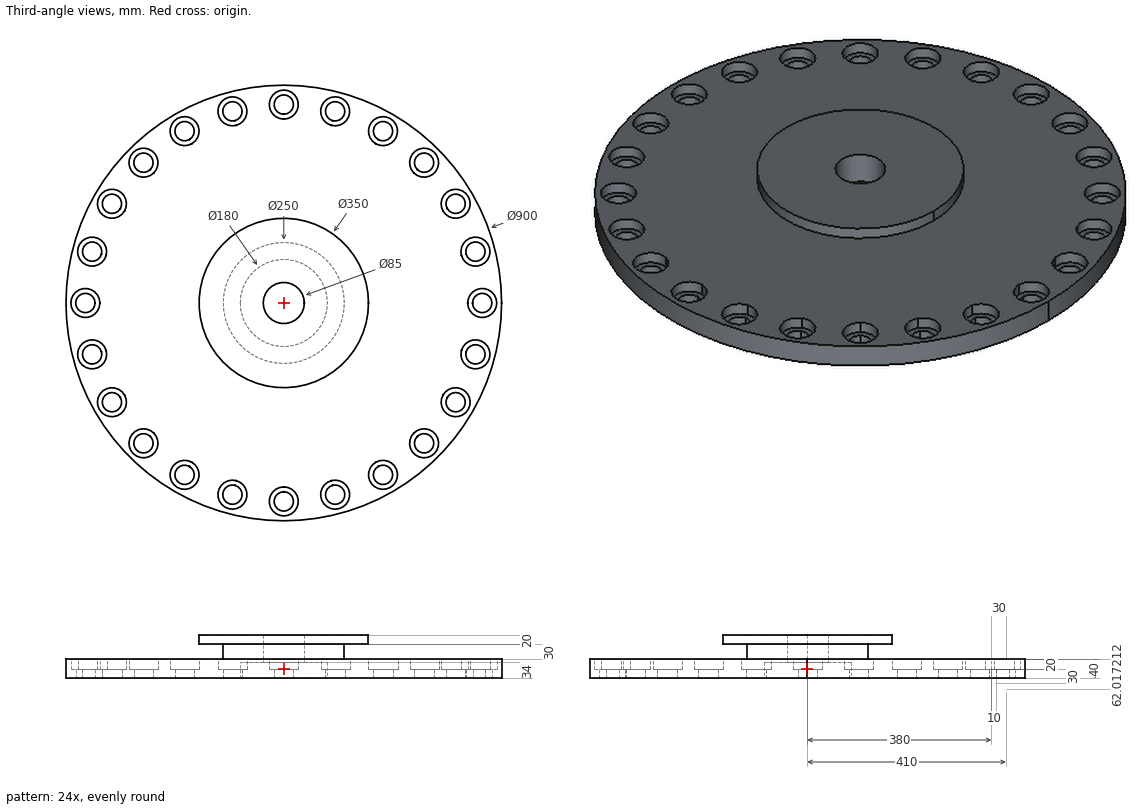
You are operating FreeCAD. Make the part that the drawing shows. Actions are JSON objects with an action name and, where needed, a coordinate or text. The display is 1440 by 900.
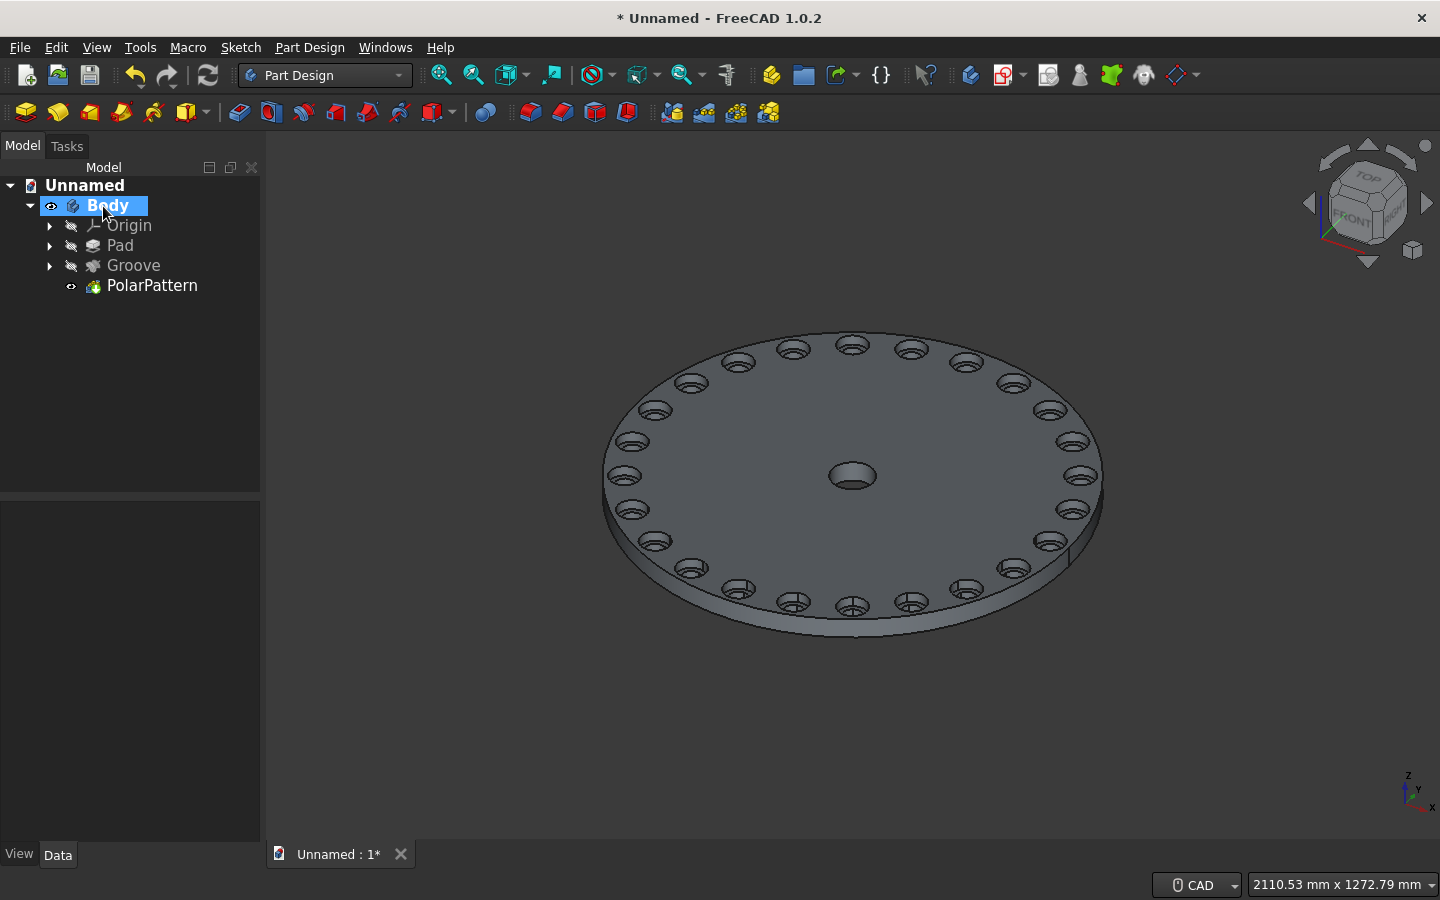
{"action": "left_click", "coordinate": [755, 490]}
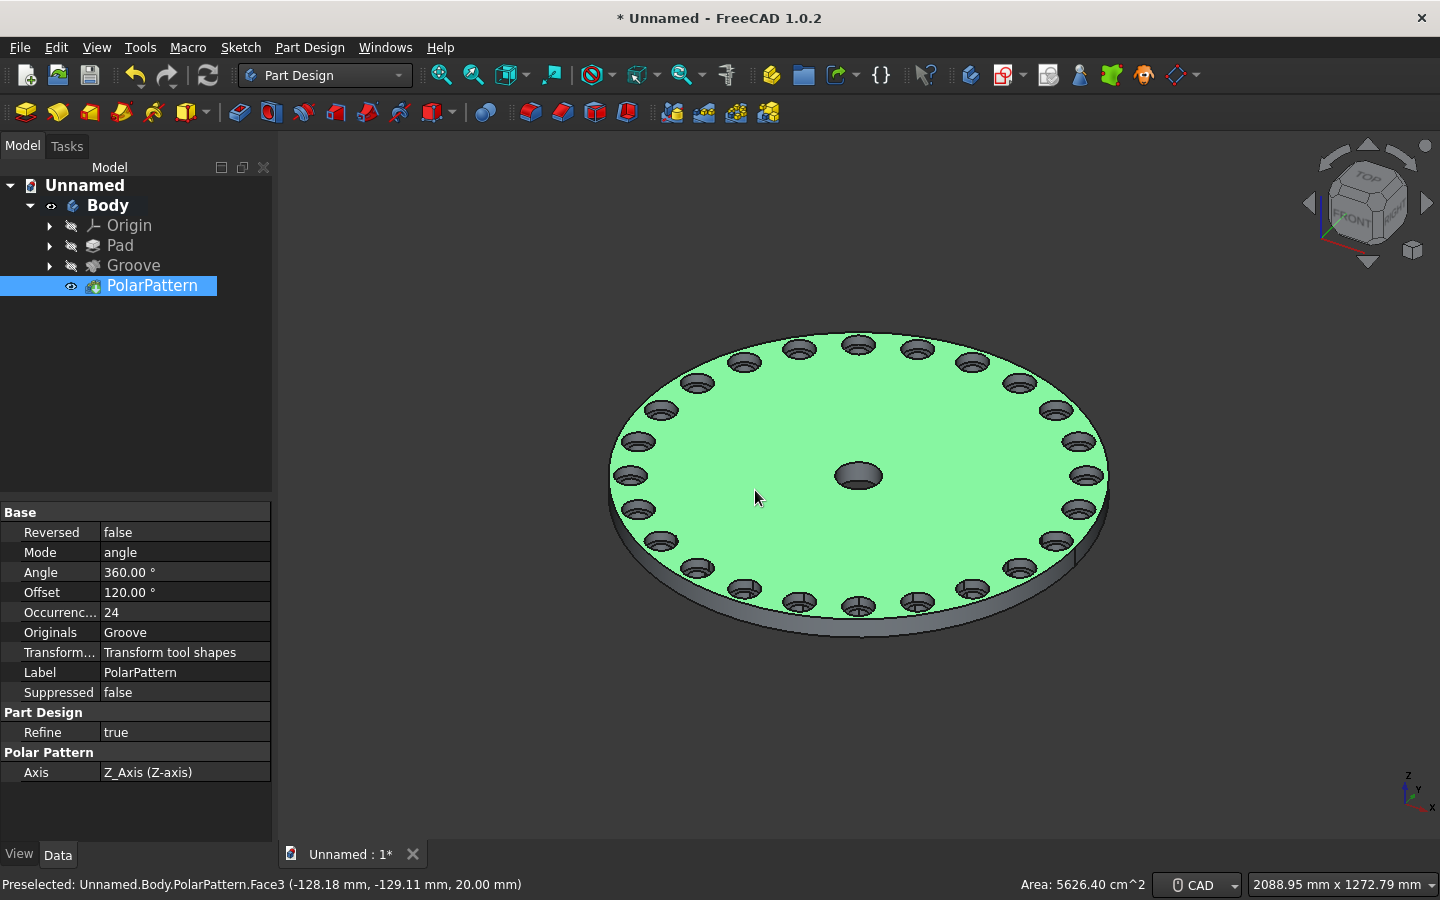
{"action": "left_click", "coordinate": [1004, 76]}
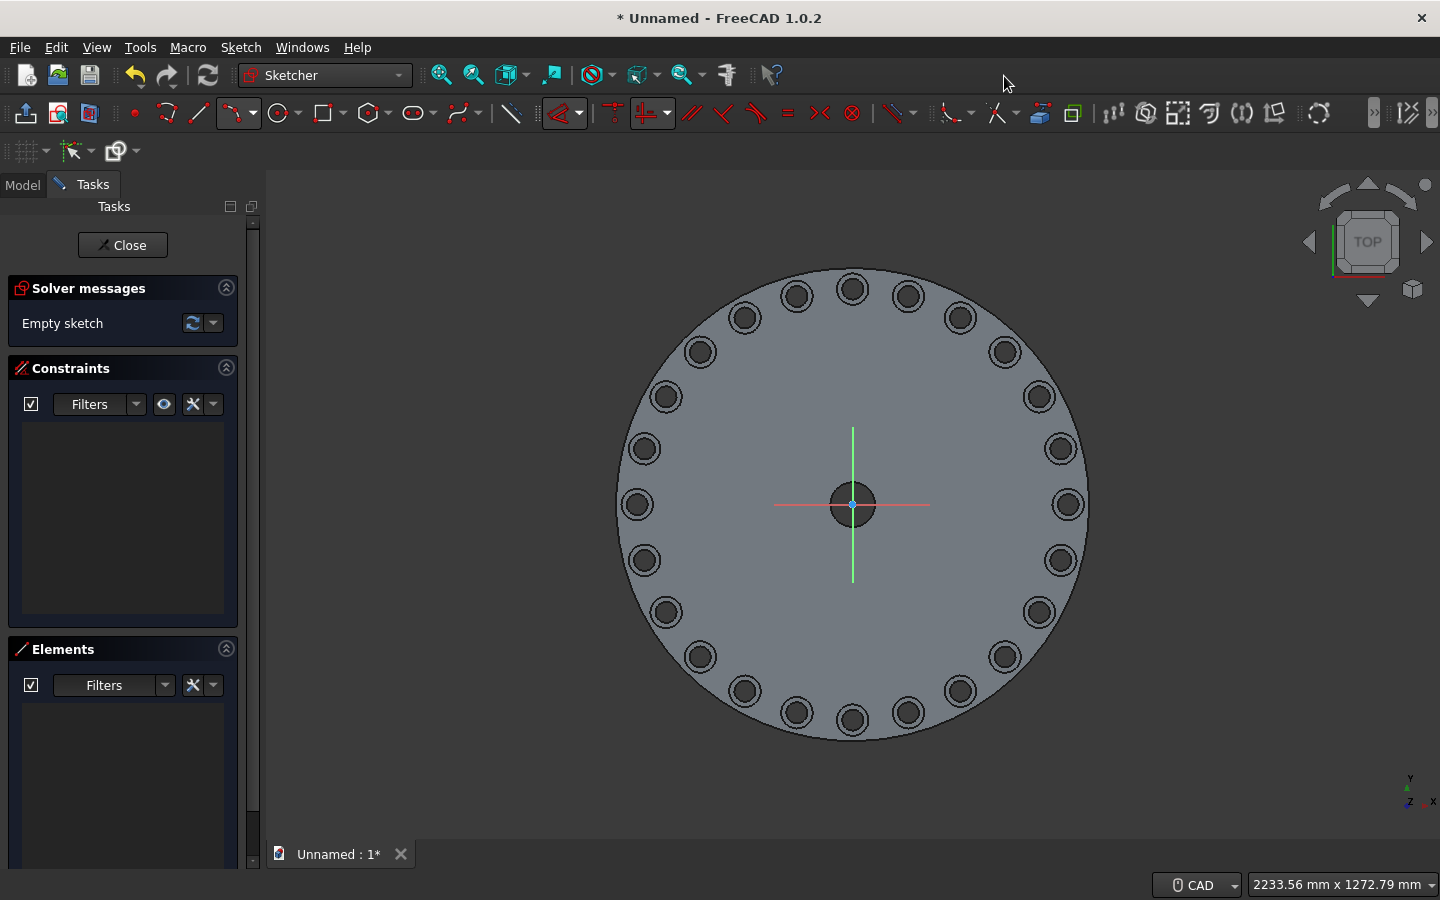
{"action": "scroll", "coordinate": [882, 505], "scroll_direction": "up", "scroll_amount": 6}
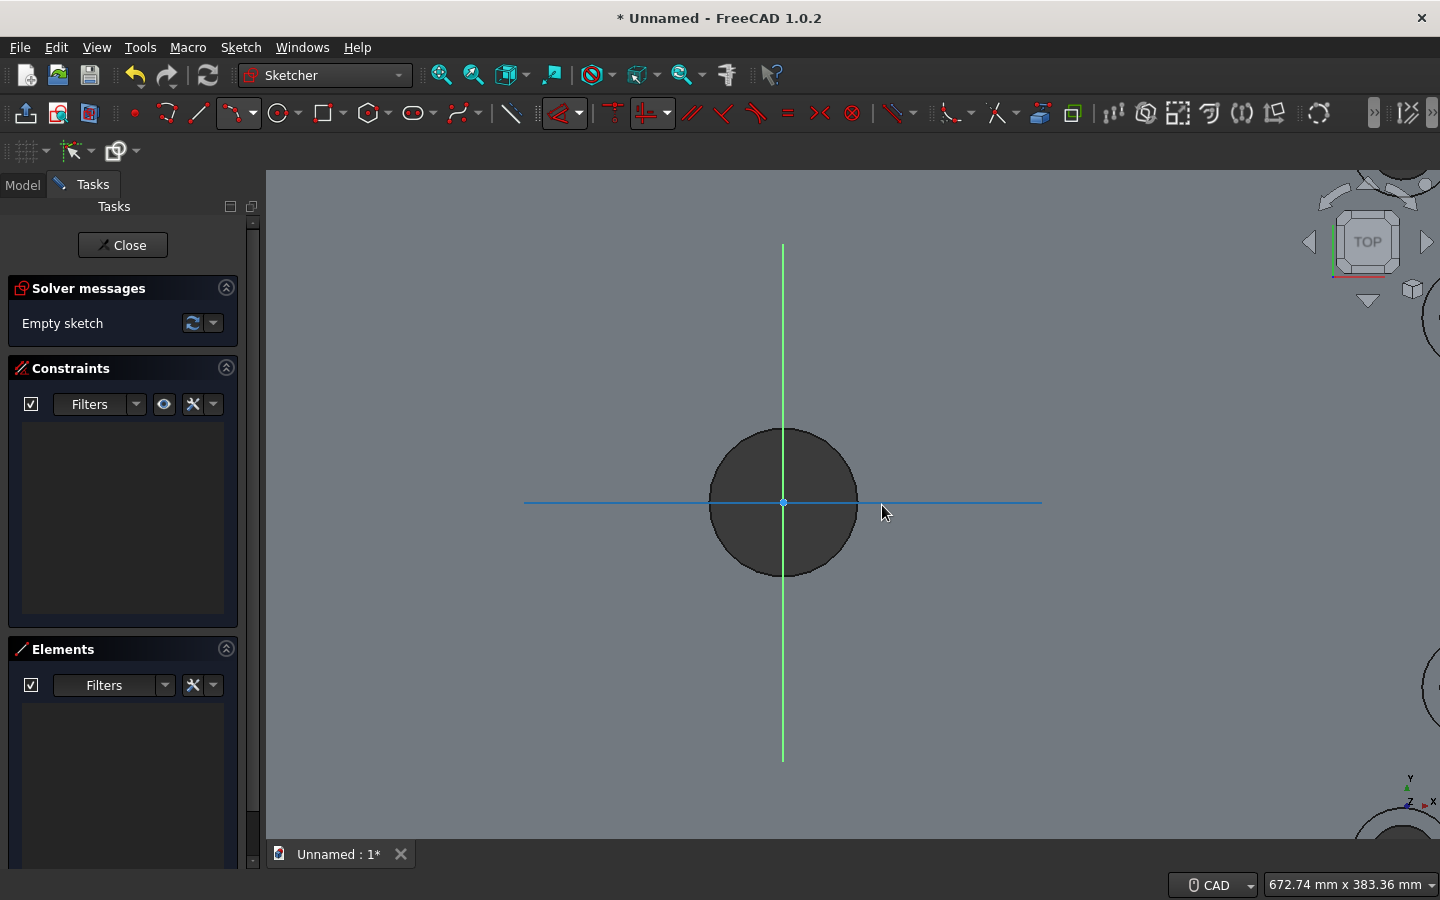
{"action": "key", "text": "g c"}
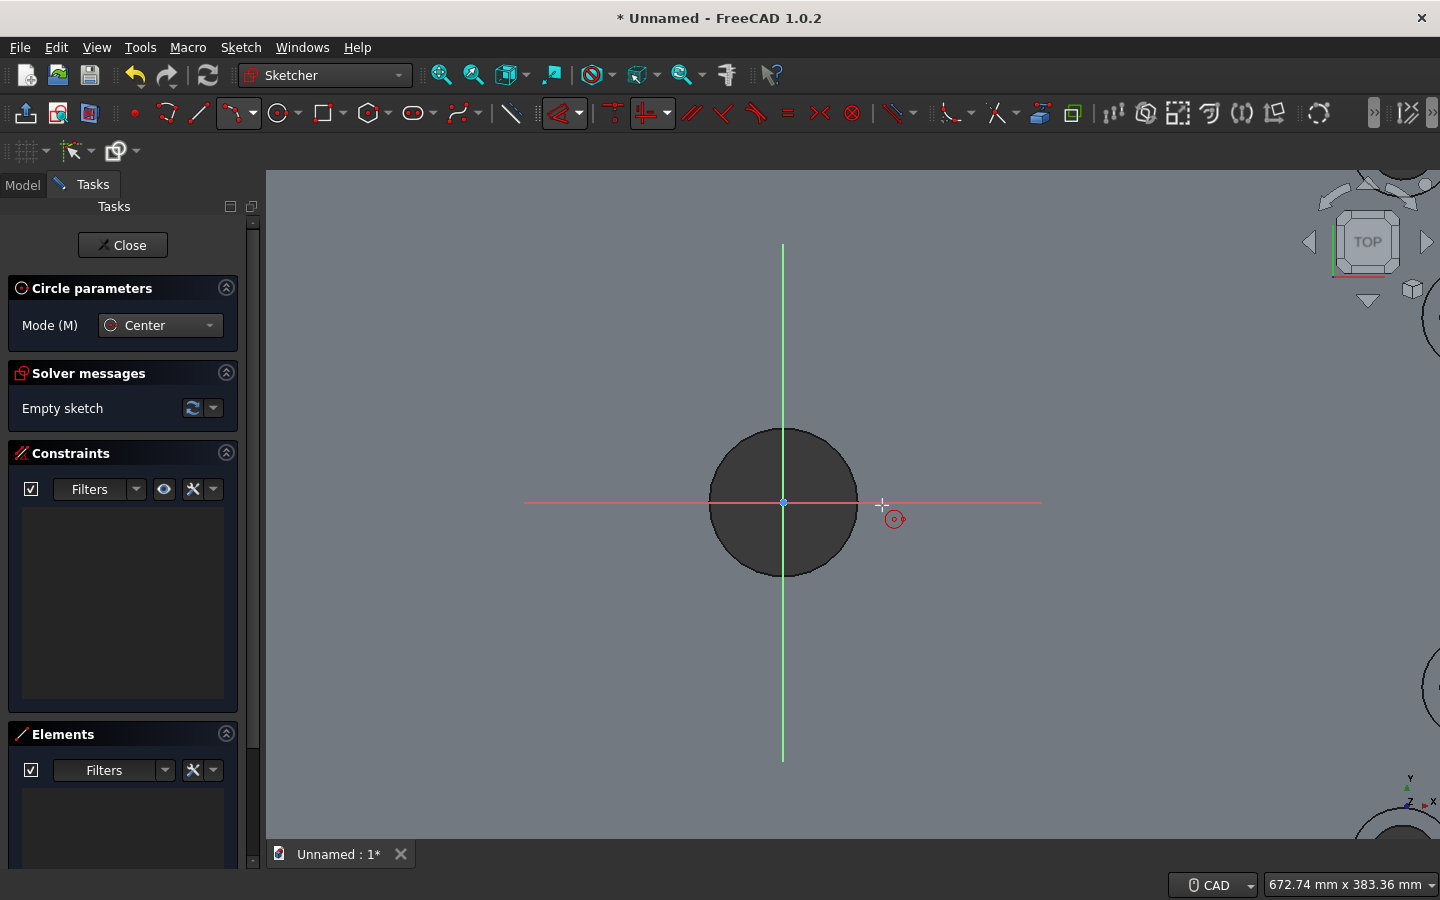
{"action": "left_click", "coordinate": [783, 503]}
{"action": "mouse_move", "coordinate": [938, 348]}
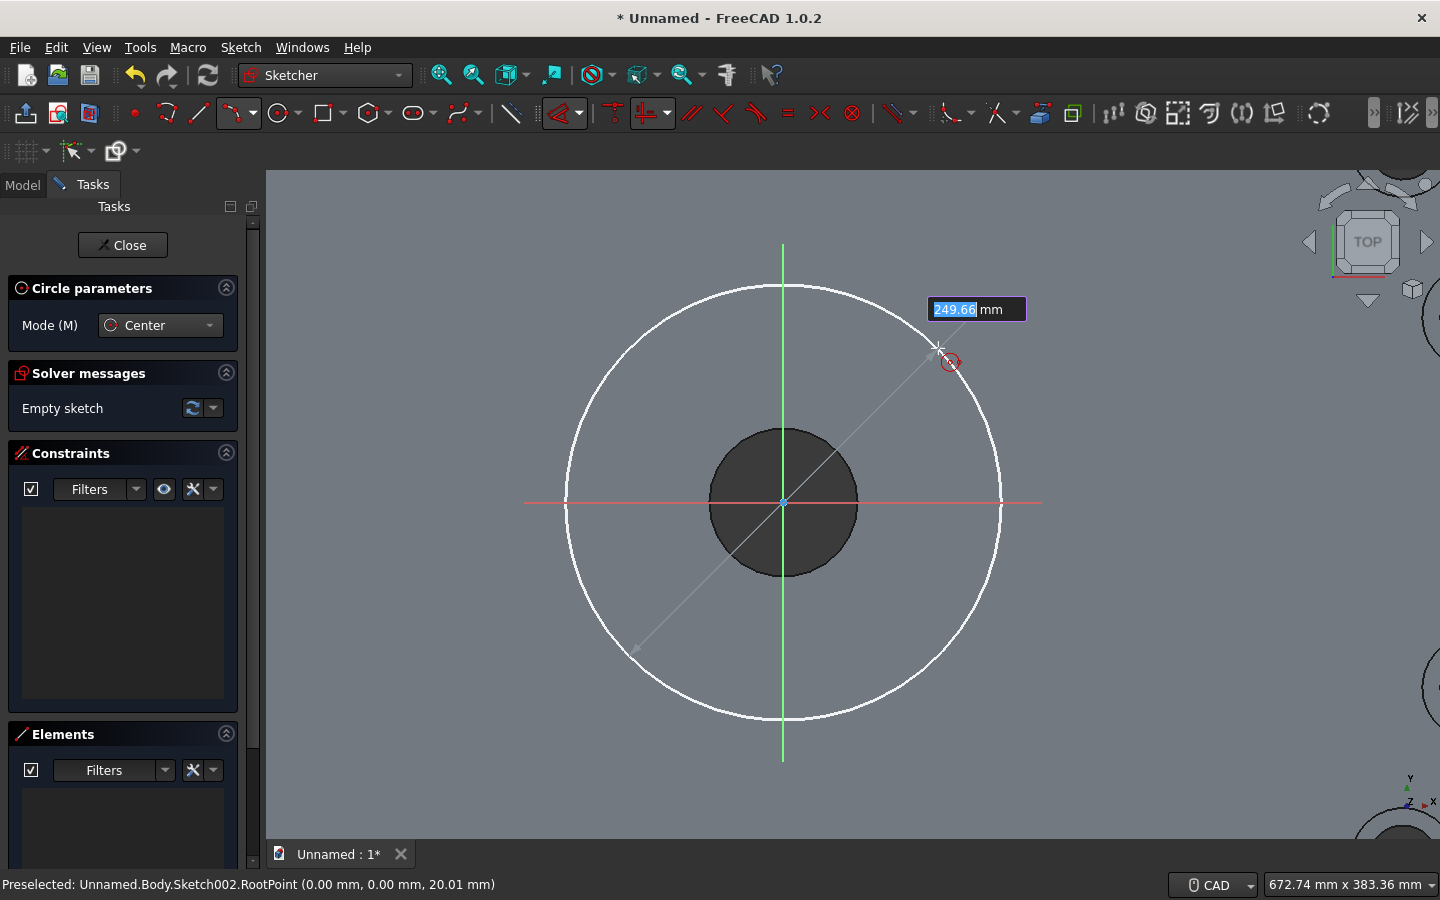
{"action": "type", "text": "250"}
{"action": "key", "text": "Return"}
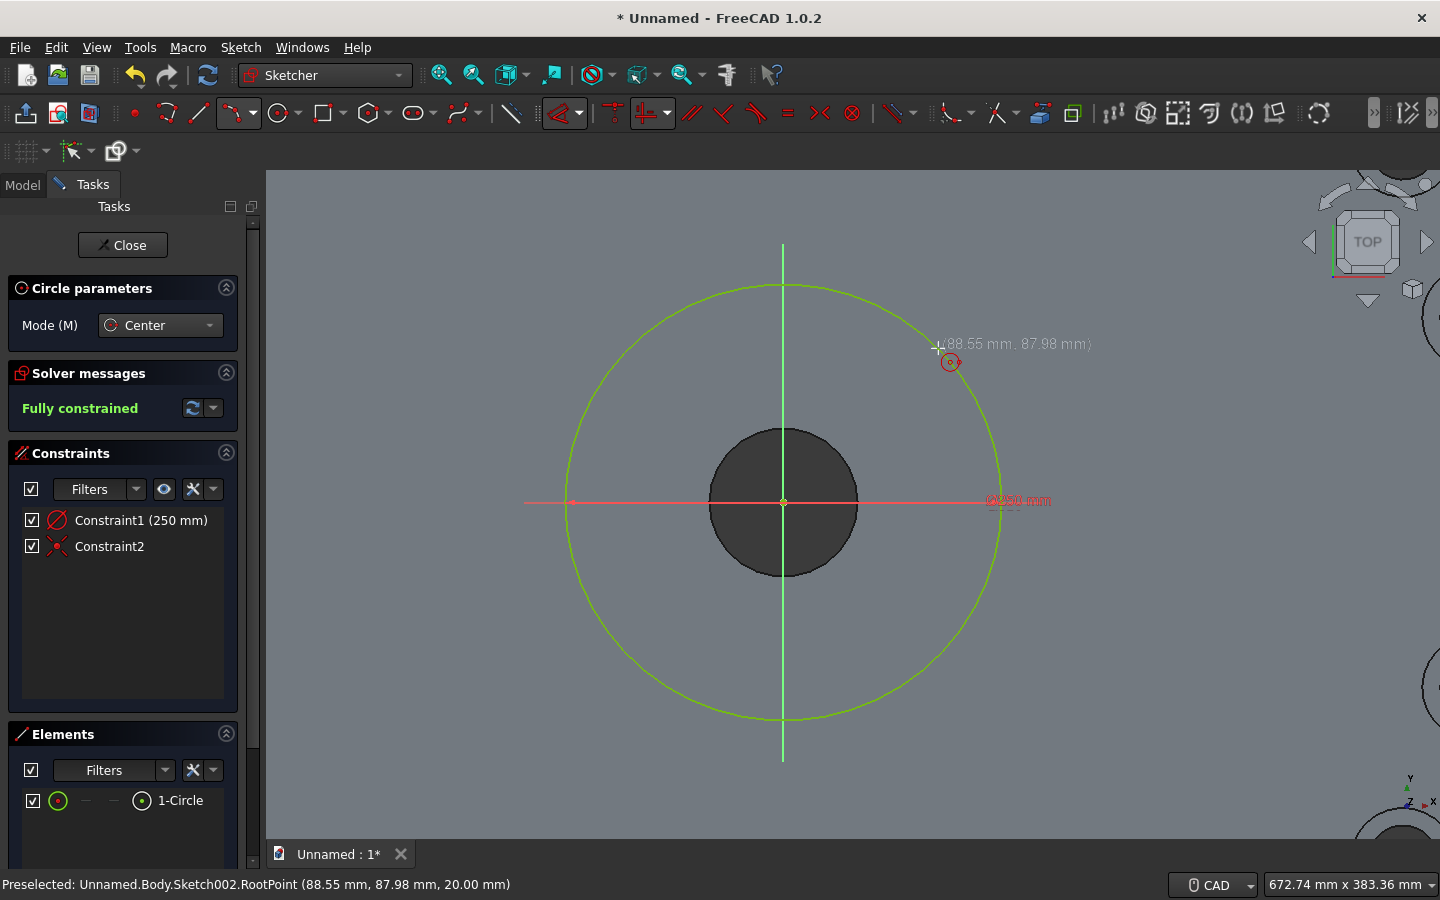
{"action": "left_click", "coordinate": [783, 503]}
{"action": "mouse_move", "coordinate": [836, 450]}